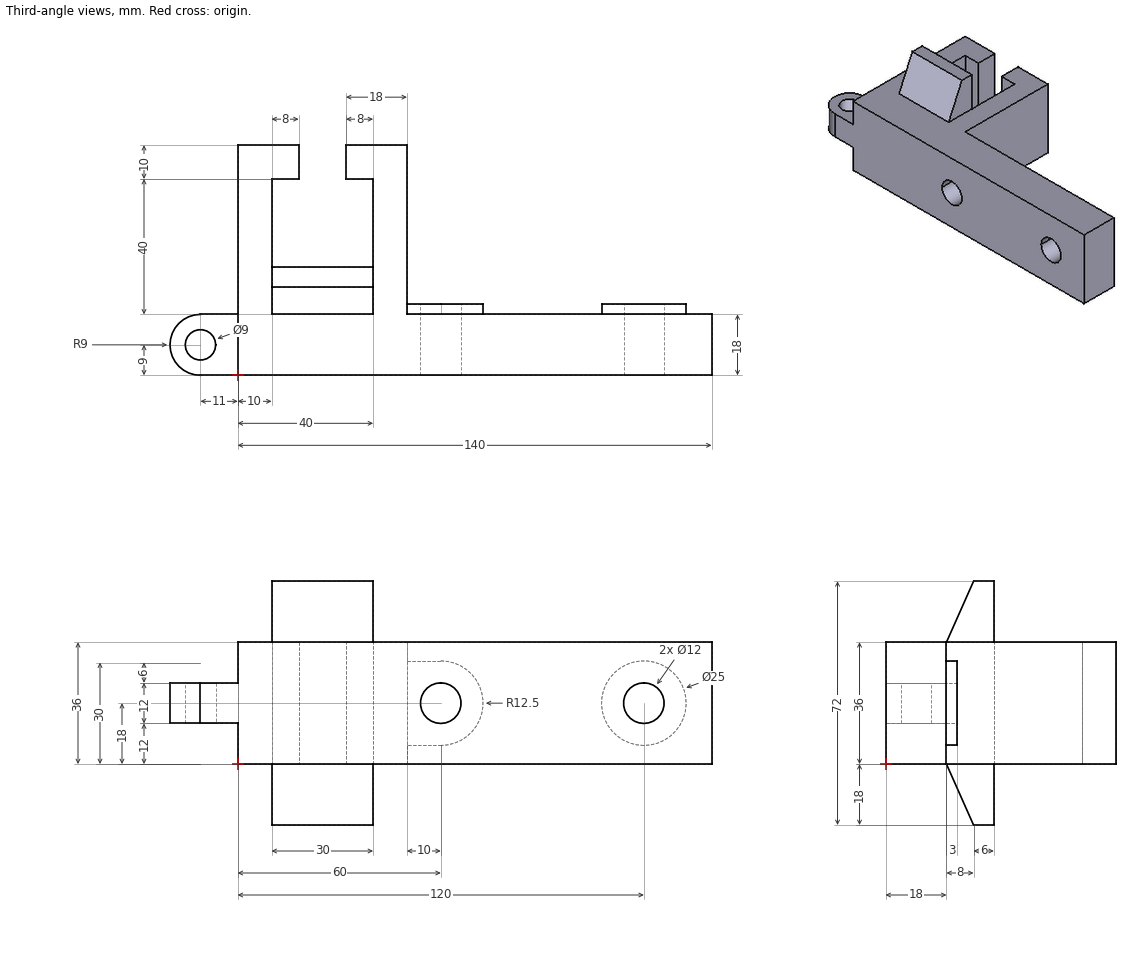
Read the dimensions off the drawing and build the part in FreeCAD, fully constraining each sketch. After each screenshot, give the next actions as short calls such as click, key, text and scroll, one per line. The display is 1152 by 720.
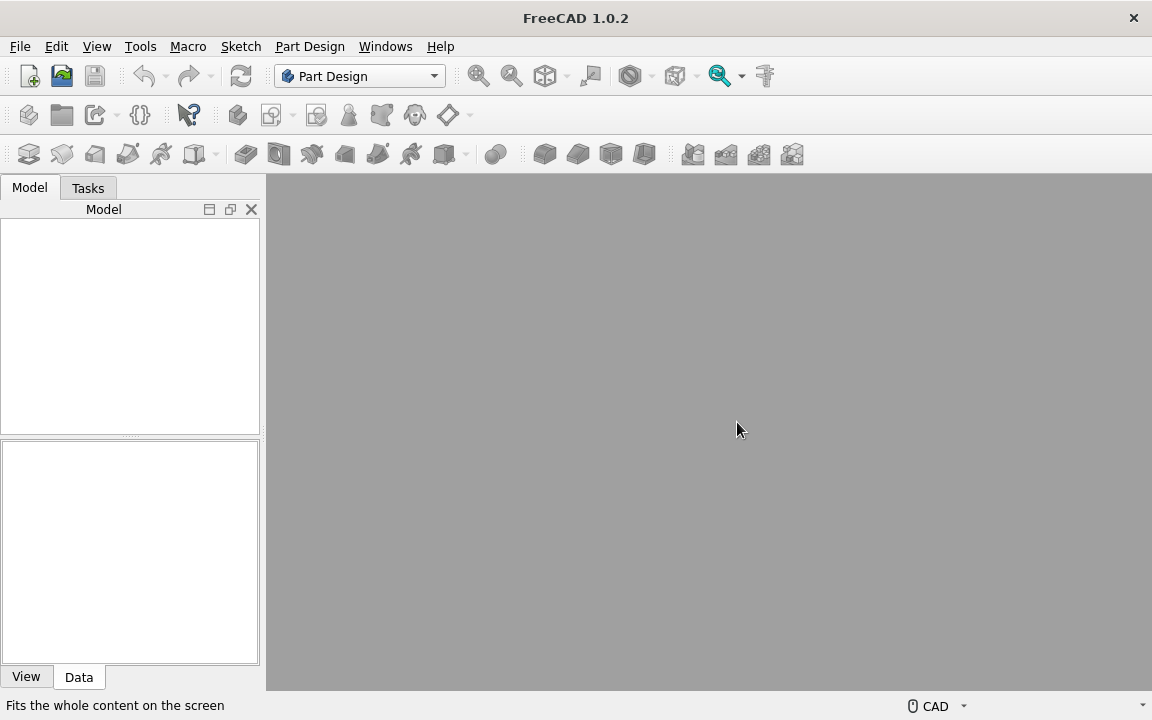
key(ctrl+n)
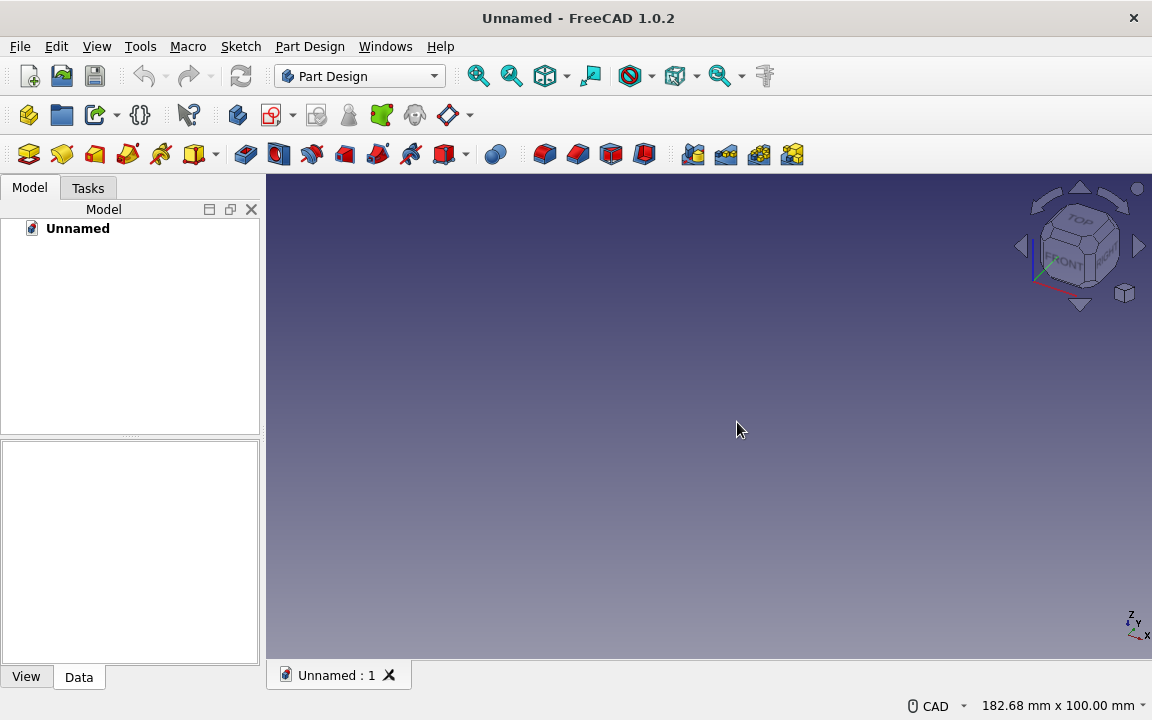
click(270, 116)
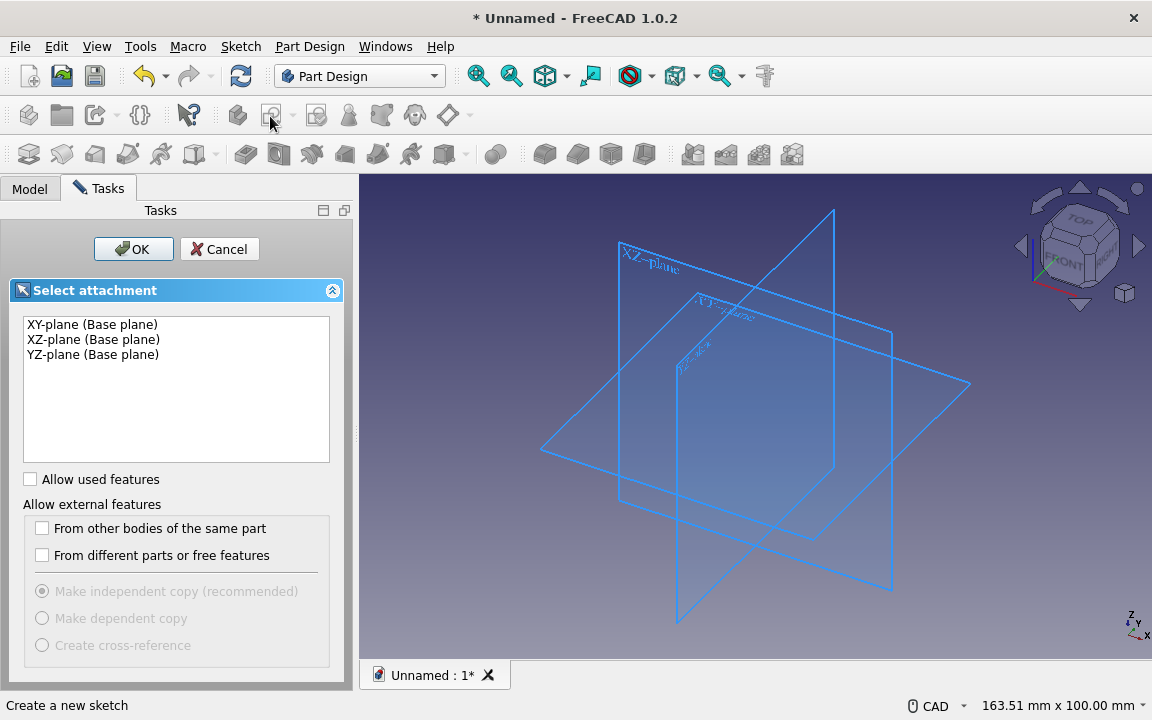
click(84, 324)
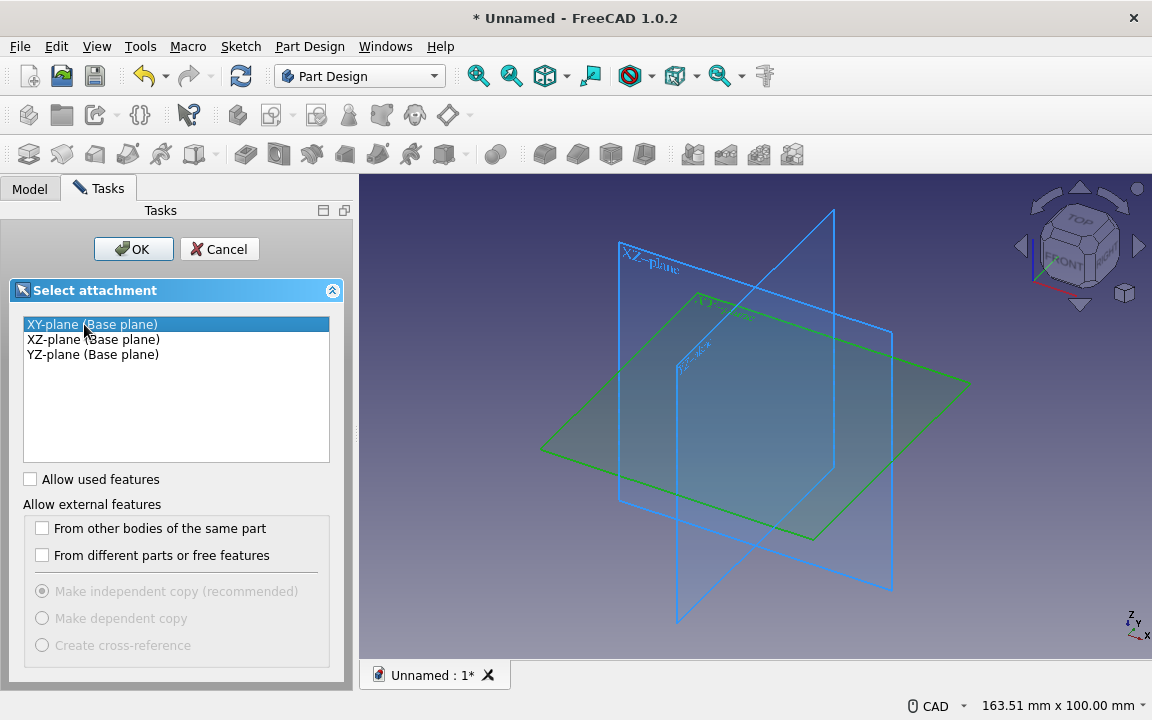
click(134, 249)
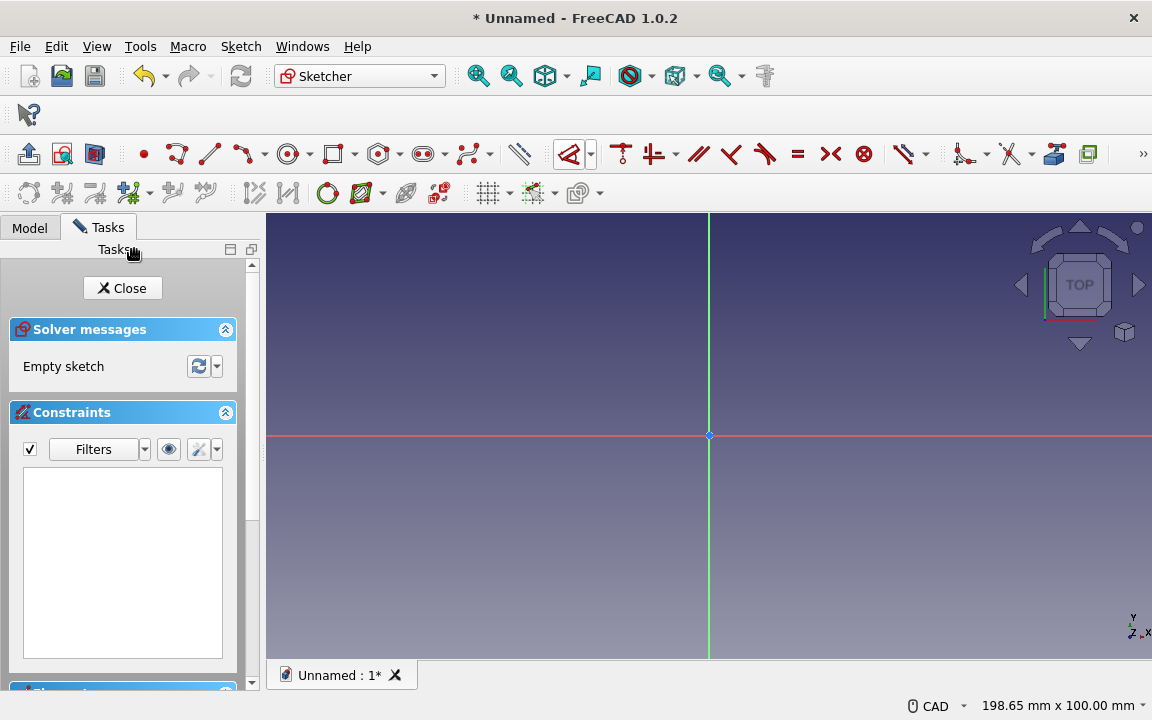
scroll(294, 485, down, 3)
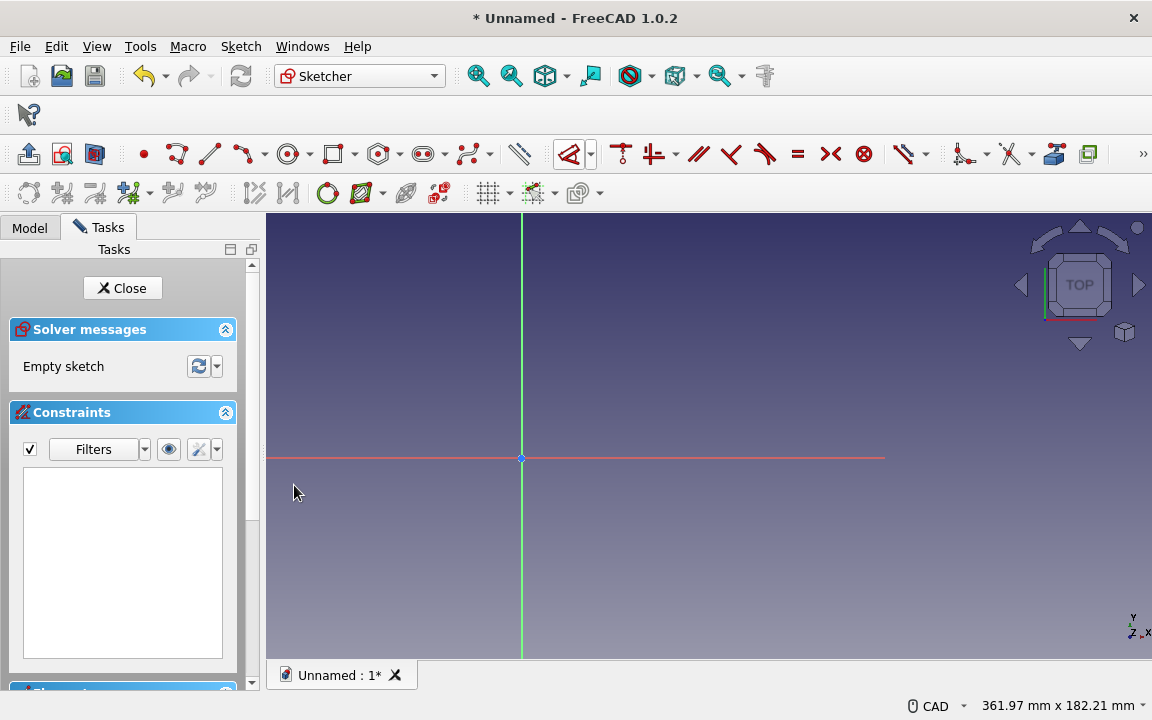
scroll(800, 437, up, 2)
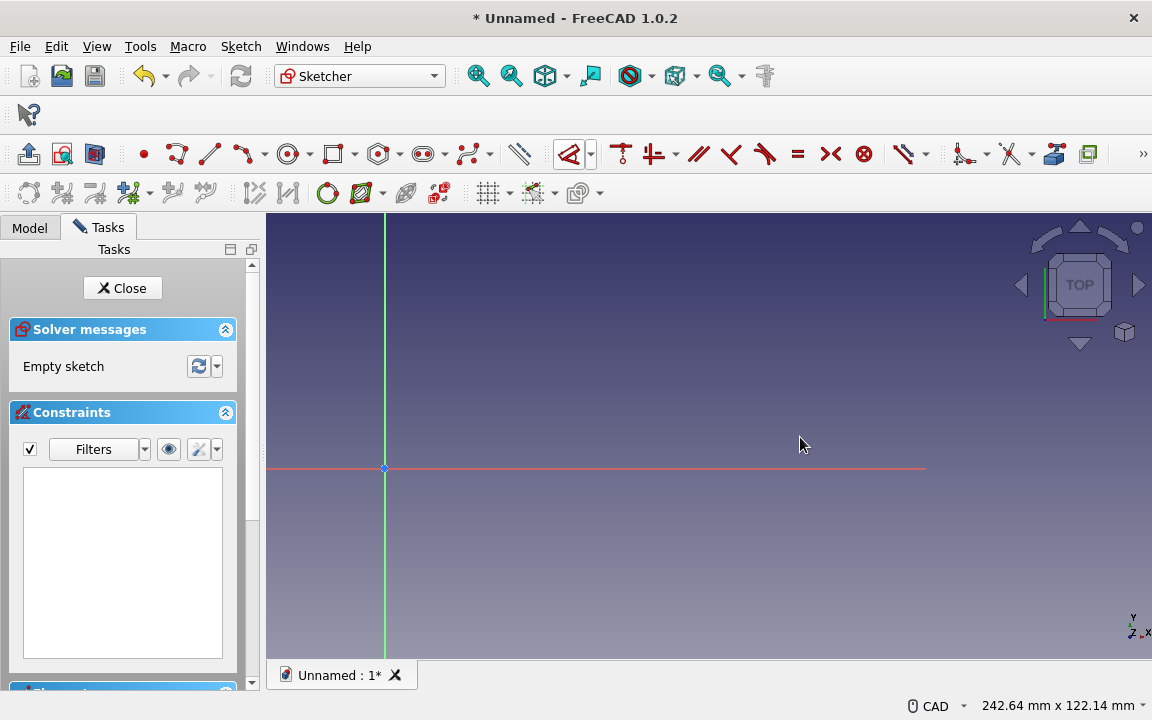
click(332, 154)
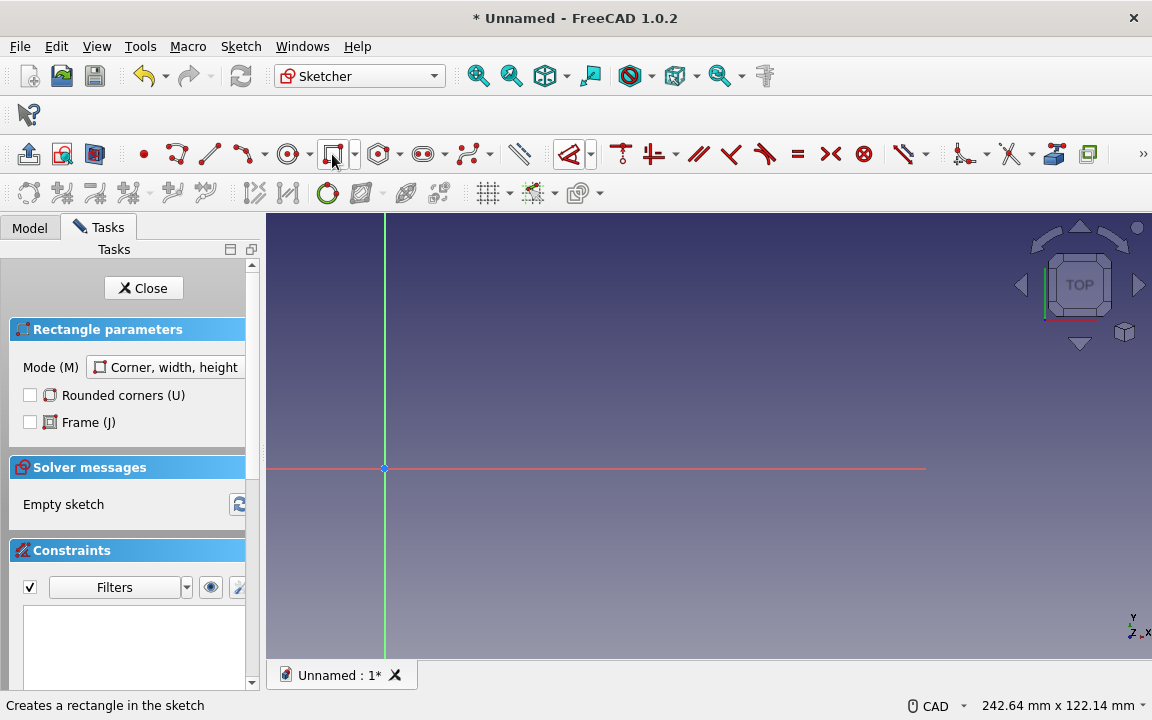
click(385, 469)
click(896, 403)
key(Escape)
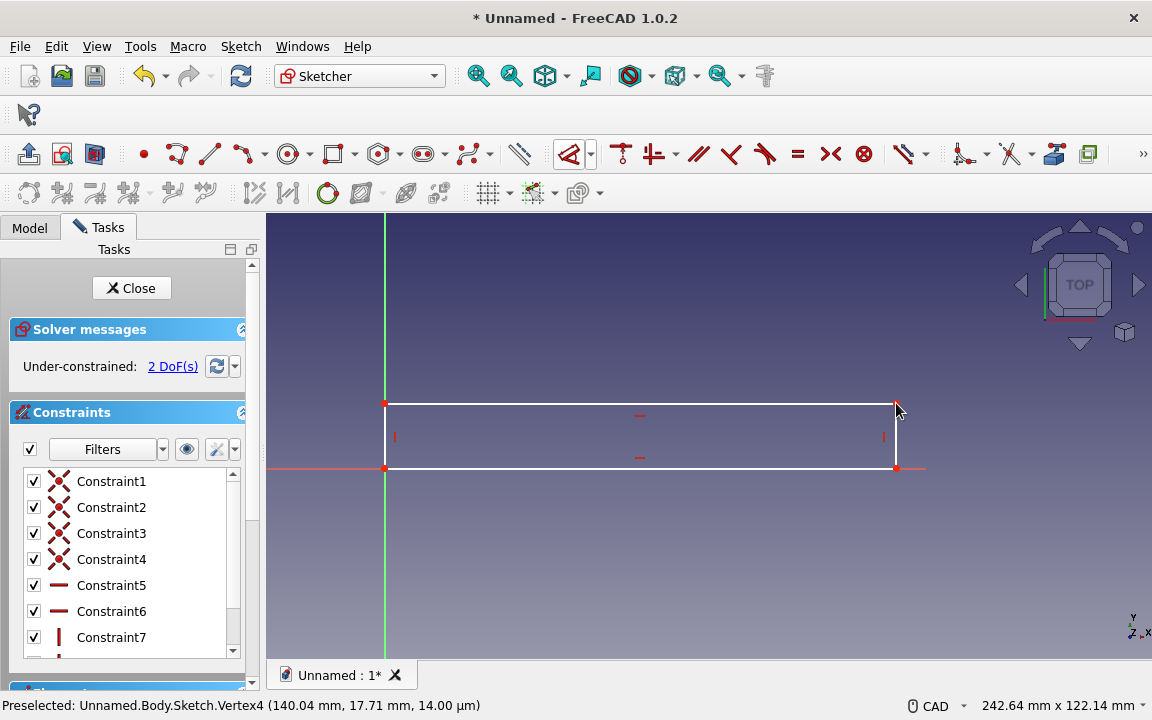
key(d)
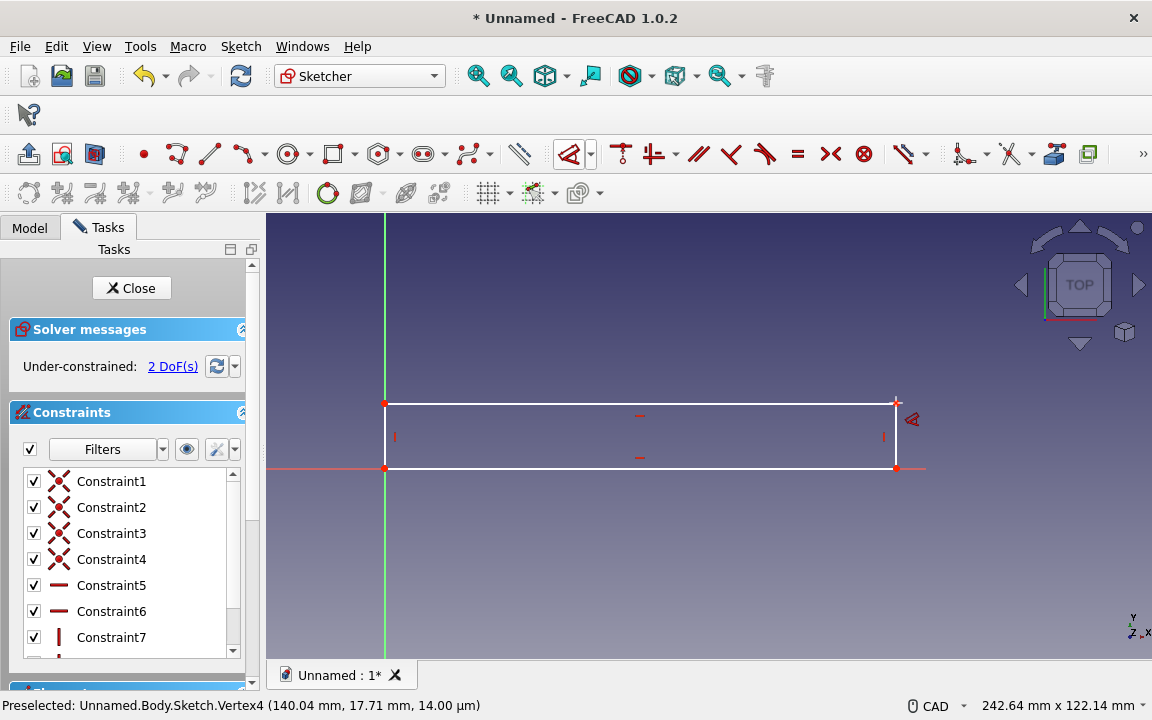
click(896, 449)
click(930, 436)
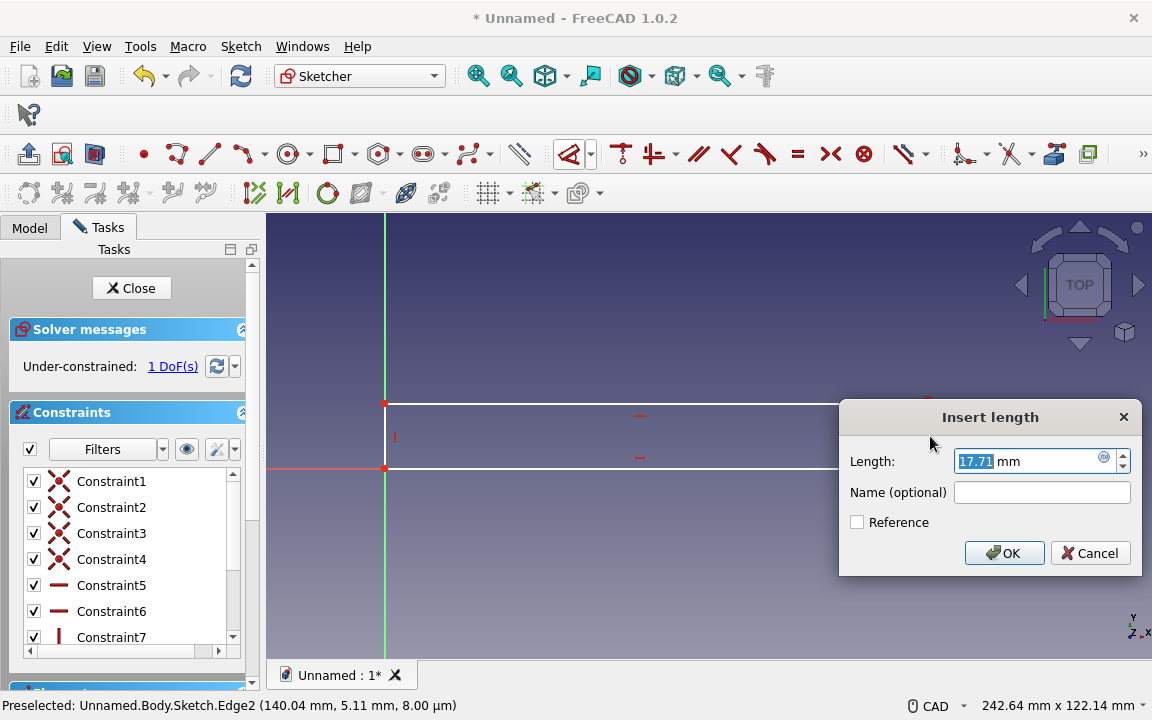
text(18)
key(Return)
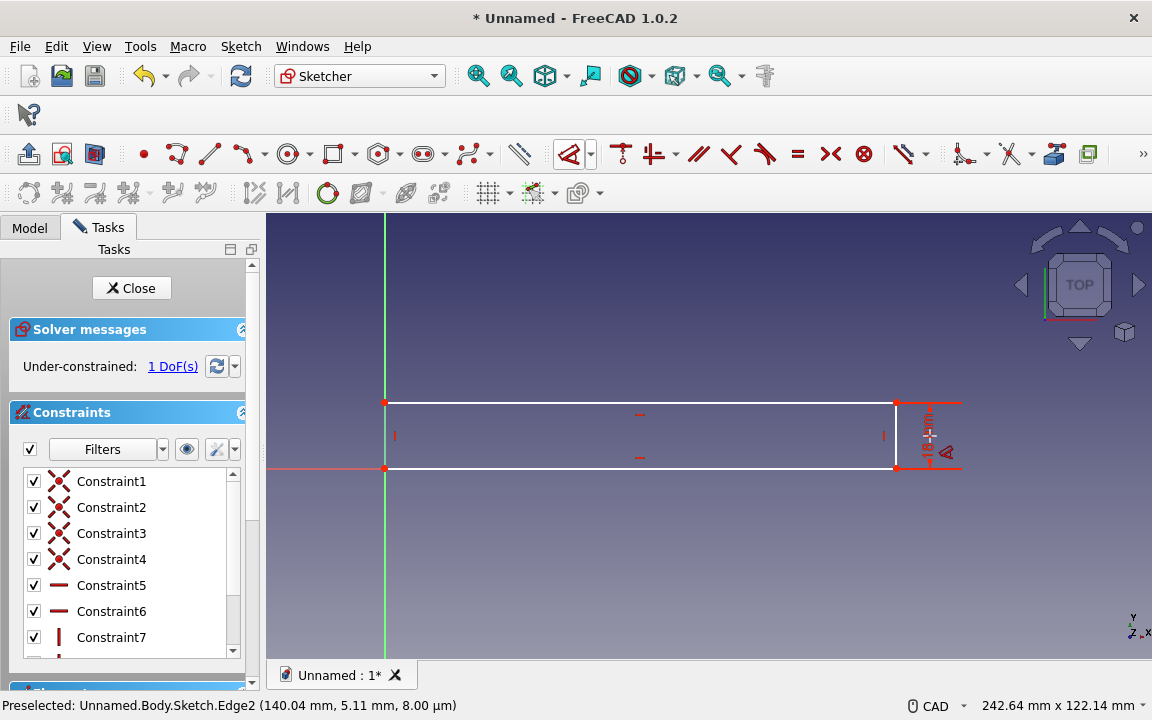
click(538, 469)
click(640, 503)